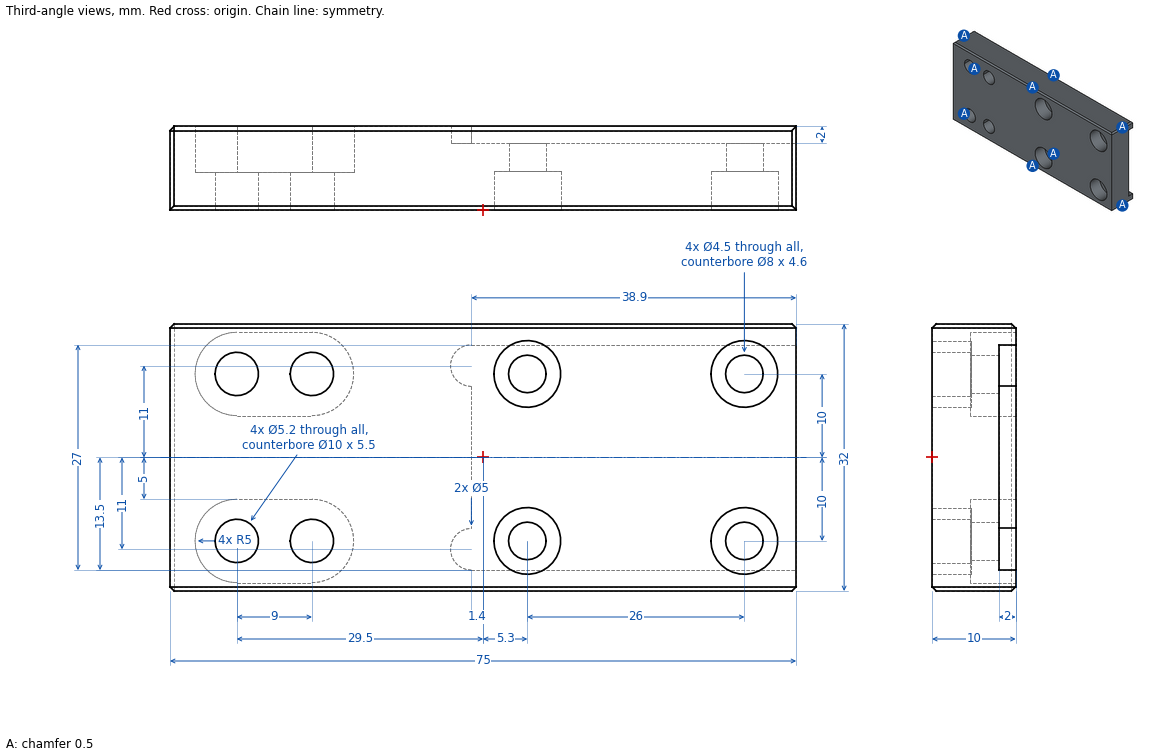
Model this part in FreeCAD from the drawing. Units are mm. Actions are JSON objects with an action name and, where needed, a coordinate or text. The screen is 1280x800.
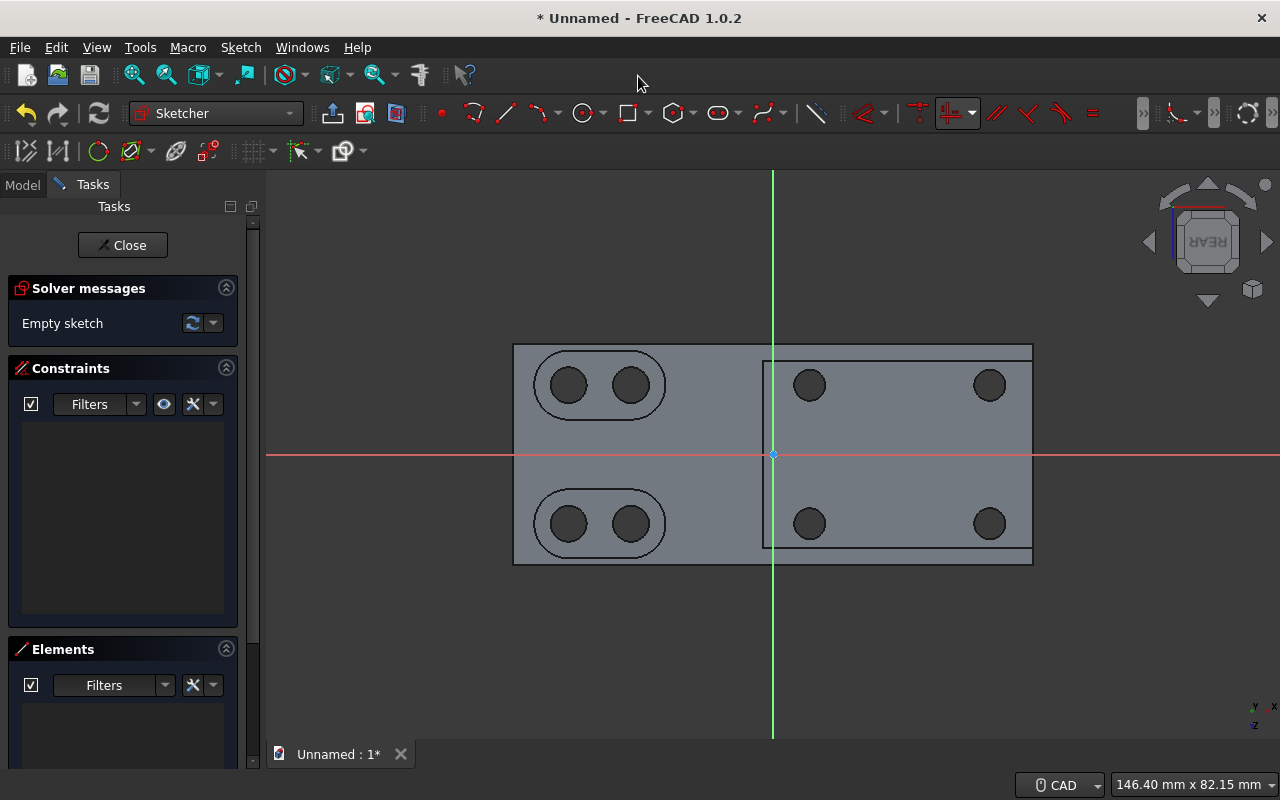
{"action": "scroll", "coordinate": [835, 454], "scroll_direction": "up", "scroll_amount": 3}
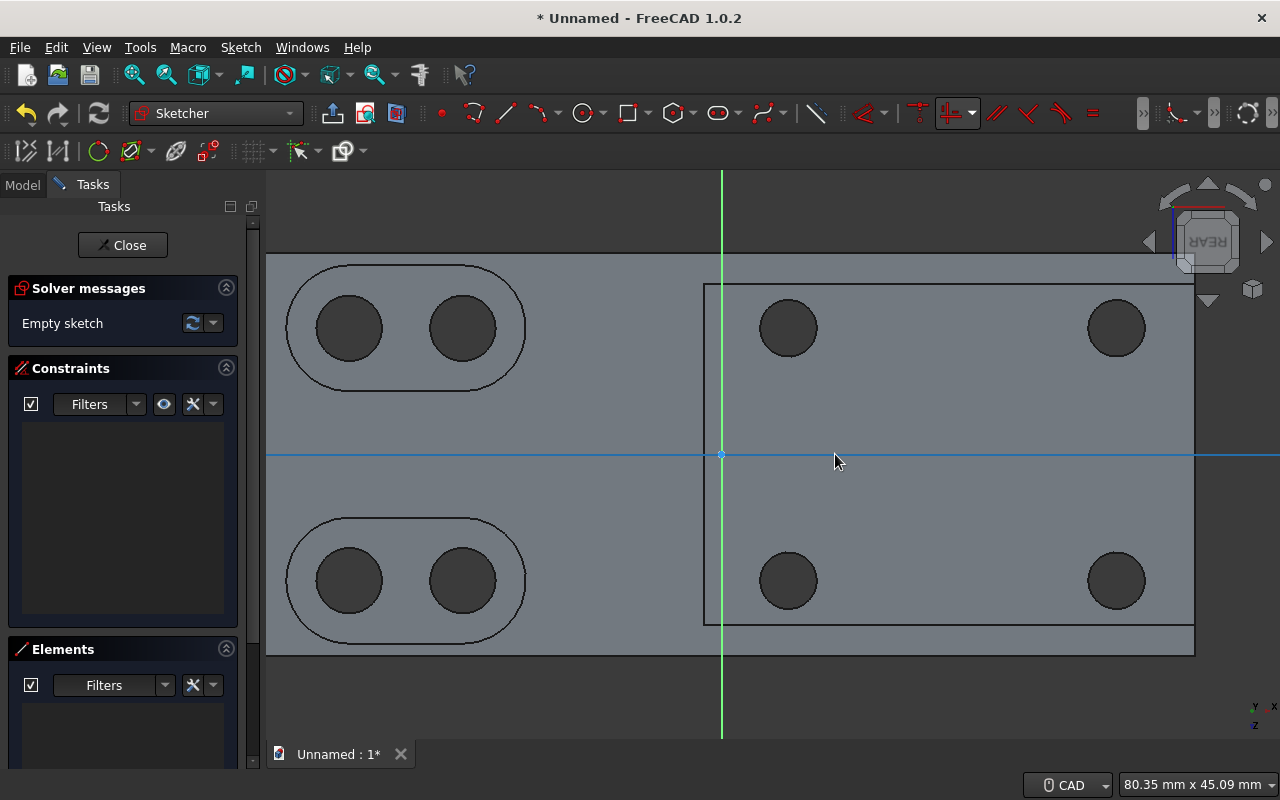
{"action": "left_click", "coordinate": [584, 114]}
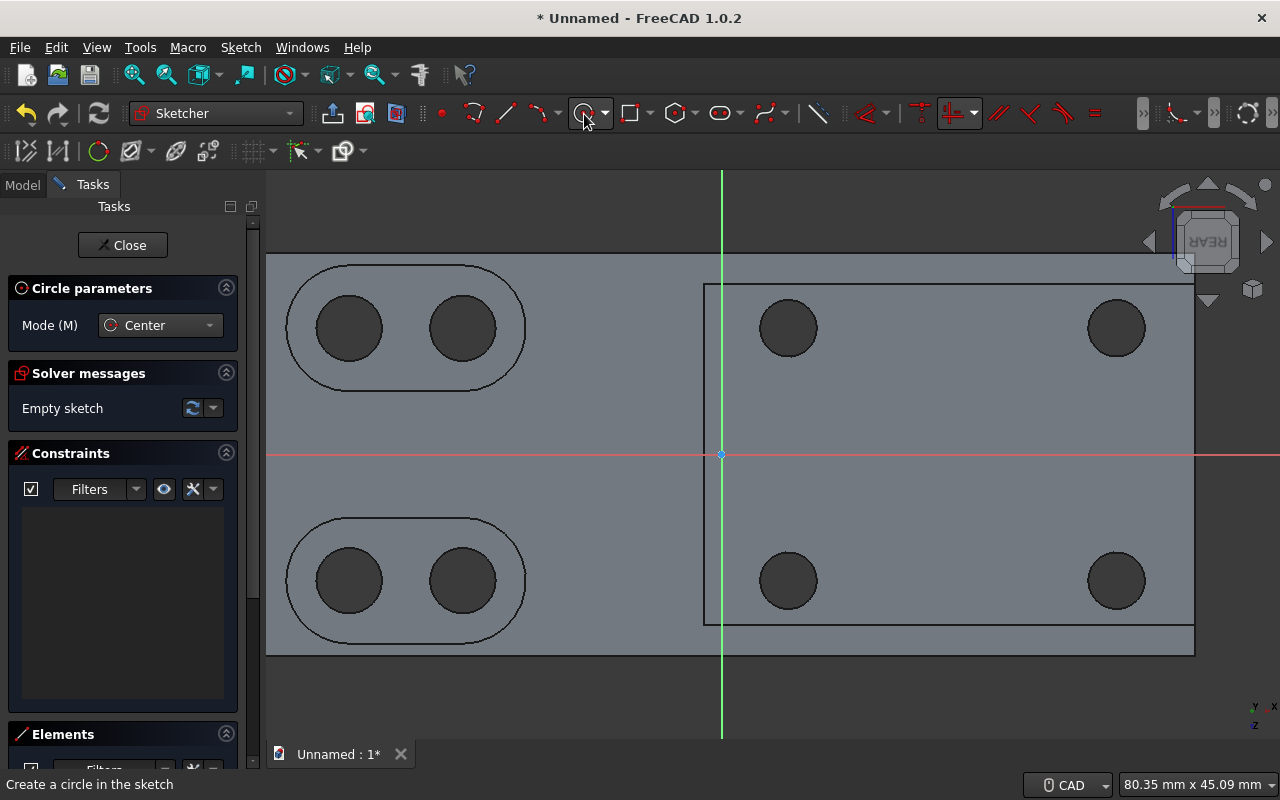
{"action": "left_click", "coordinate": [704, 316]}
{"action": "left_click", "coordinate": [682, 293]}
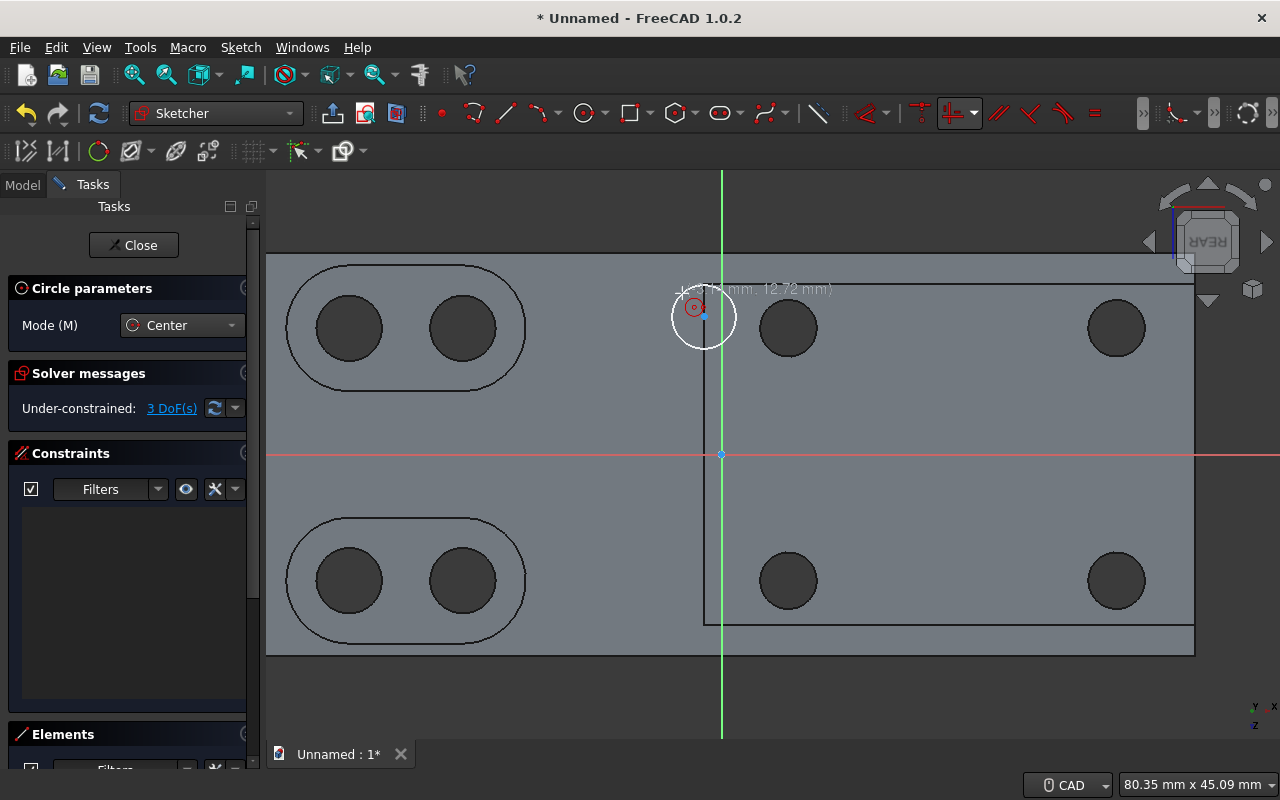
{"action": "left_click", "coordinate": [704, 593]}
{"action": "left_click", "coordinate": [682, 571]}
{"action": "key", "text": "Escape"}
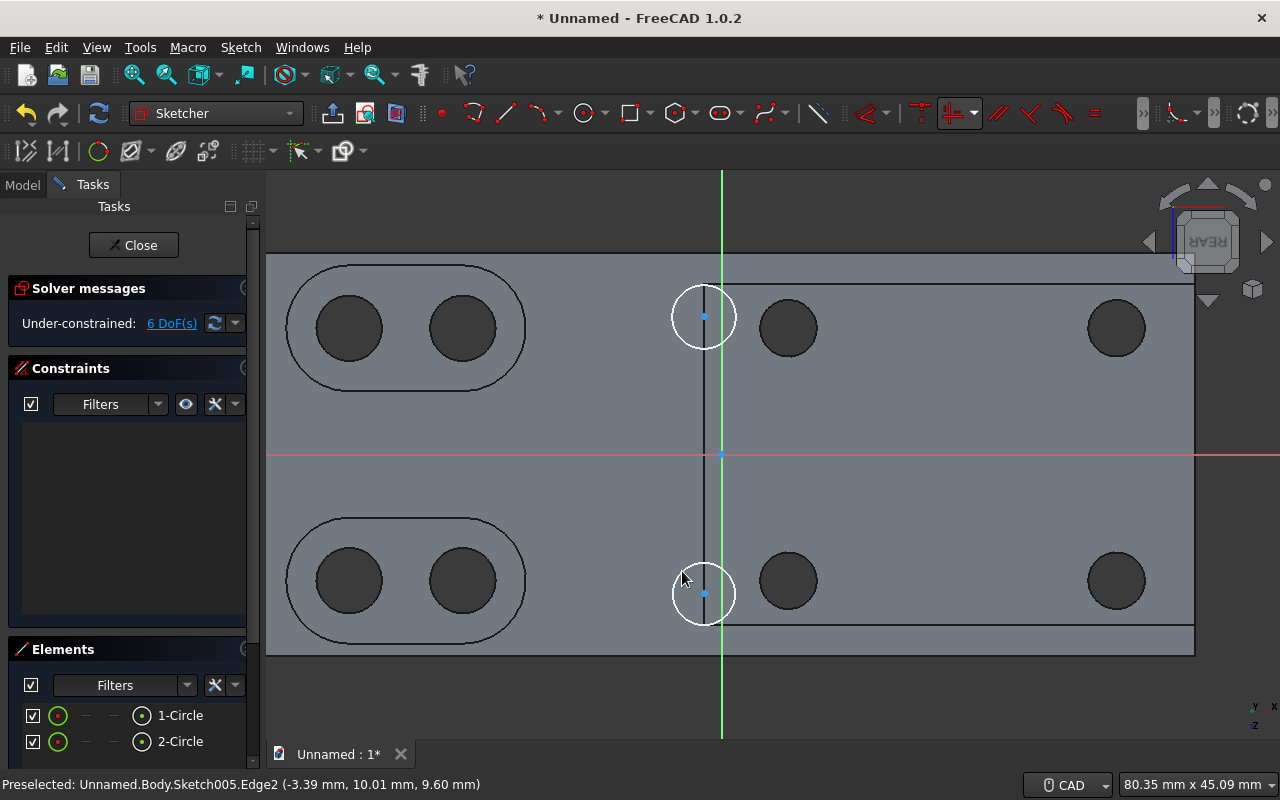
{"action": "left_click", "coordinate": [681, 295]}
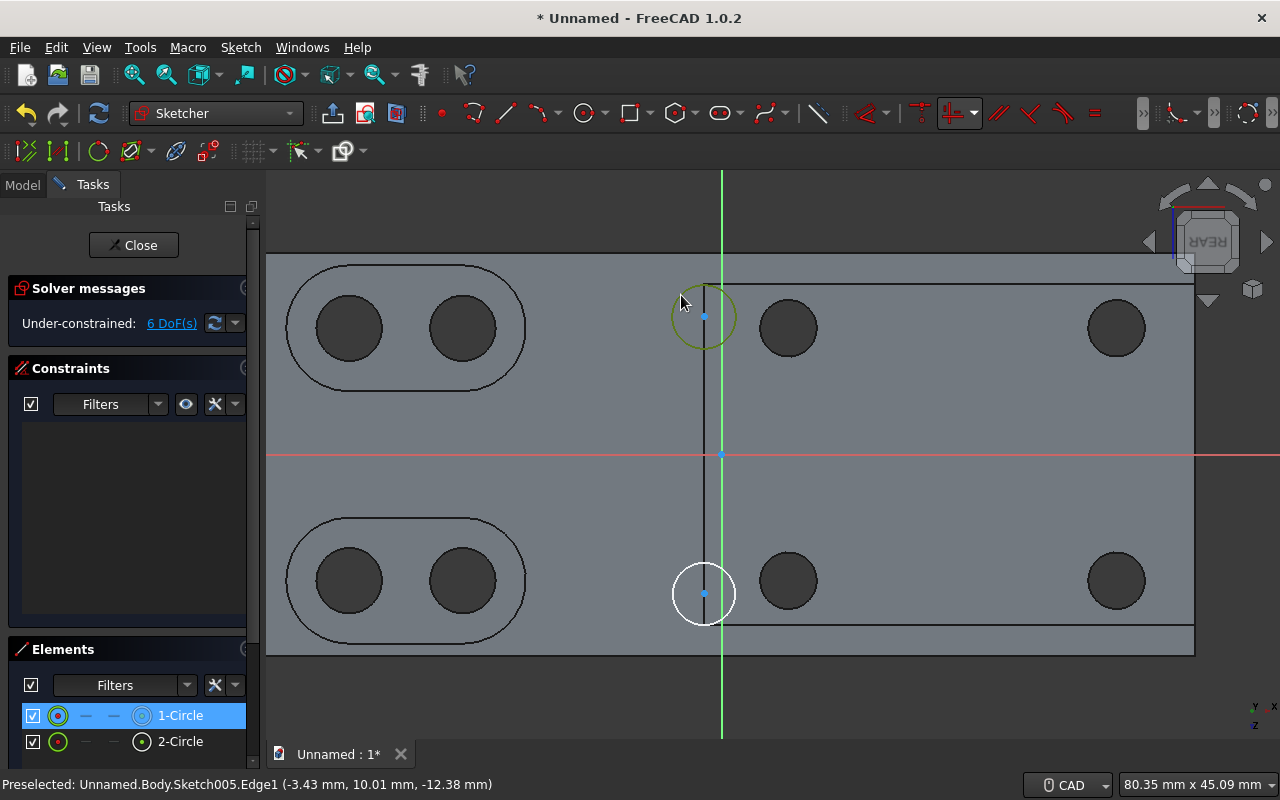
{"action": "left_click", "coordinate": [682, 572]}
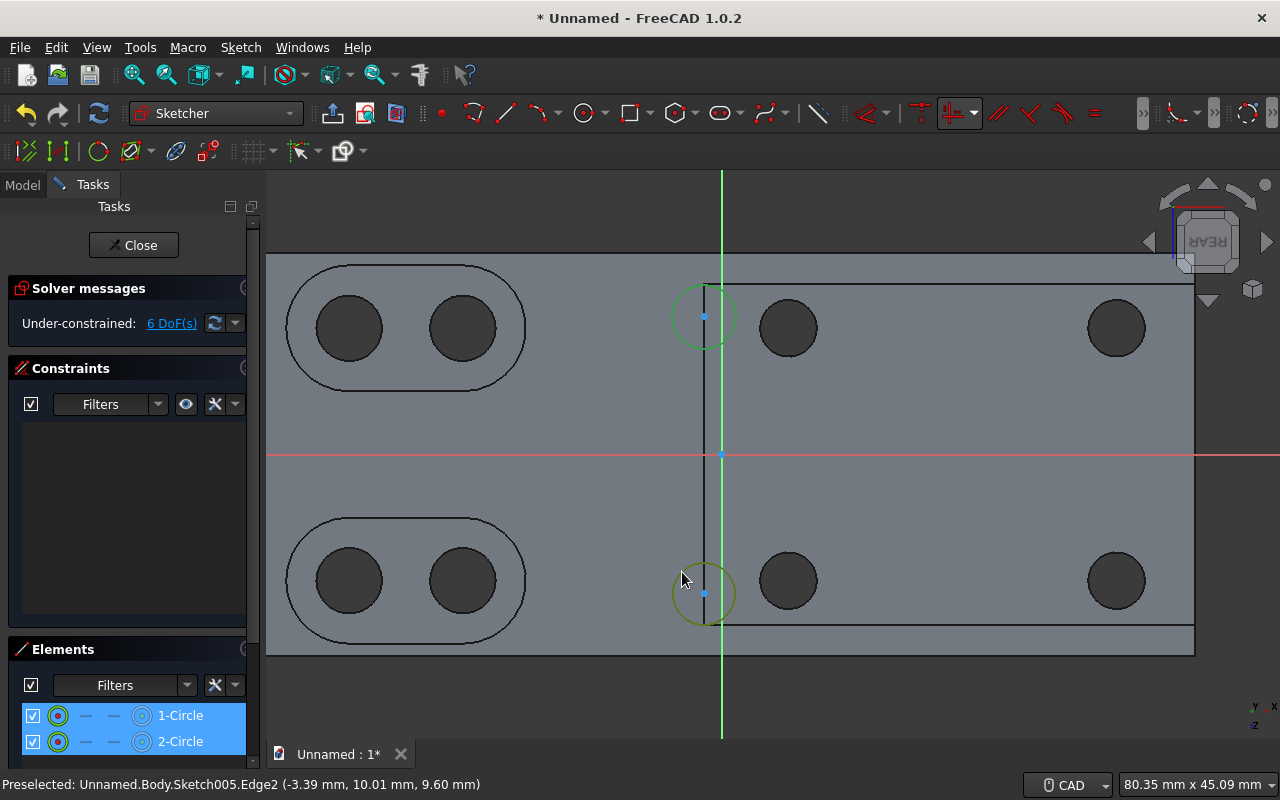
{"action": "left_click", "coordinate": [1096, 114]}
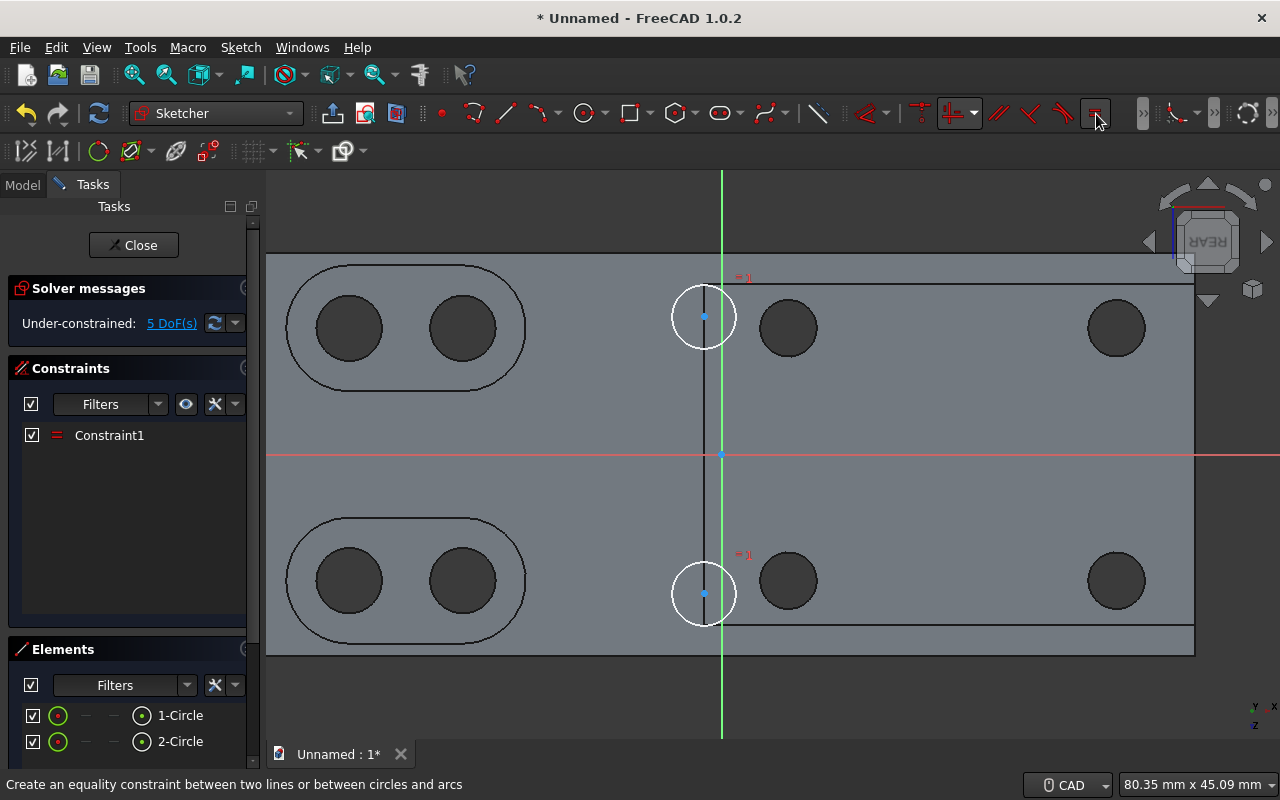
{"action": "left_click", "coordinate": [704, 317]}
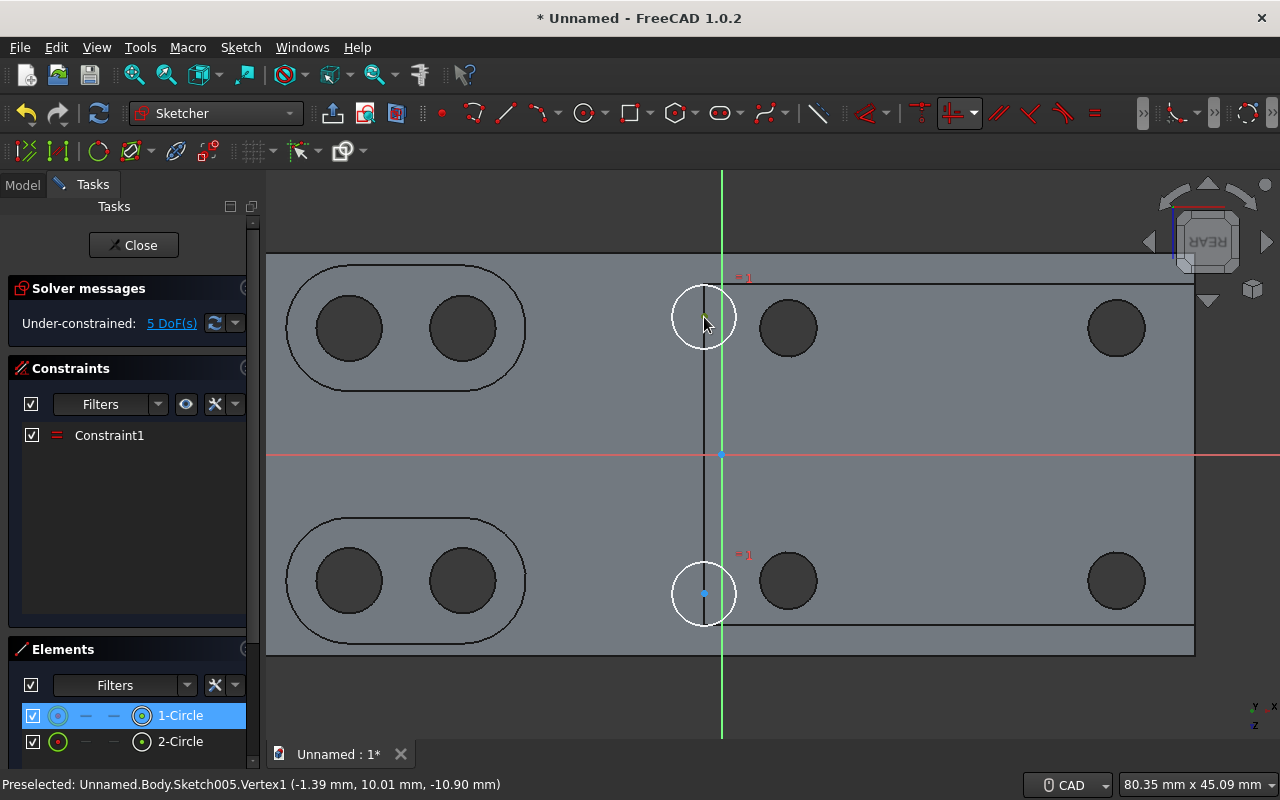
{"action": "left_click", "coordinate": [704, 594]}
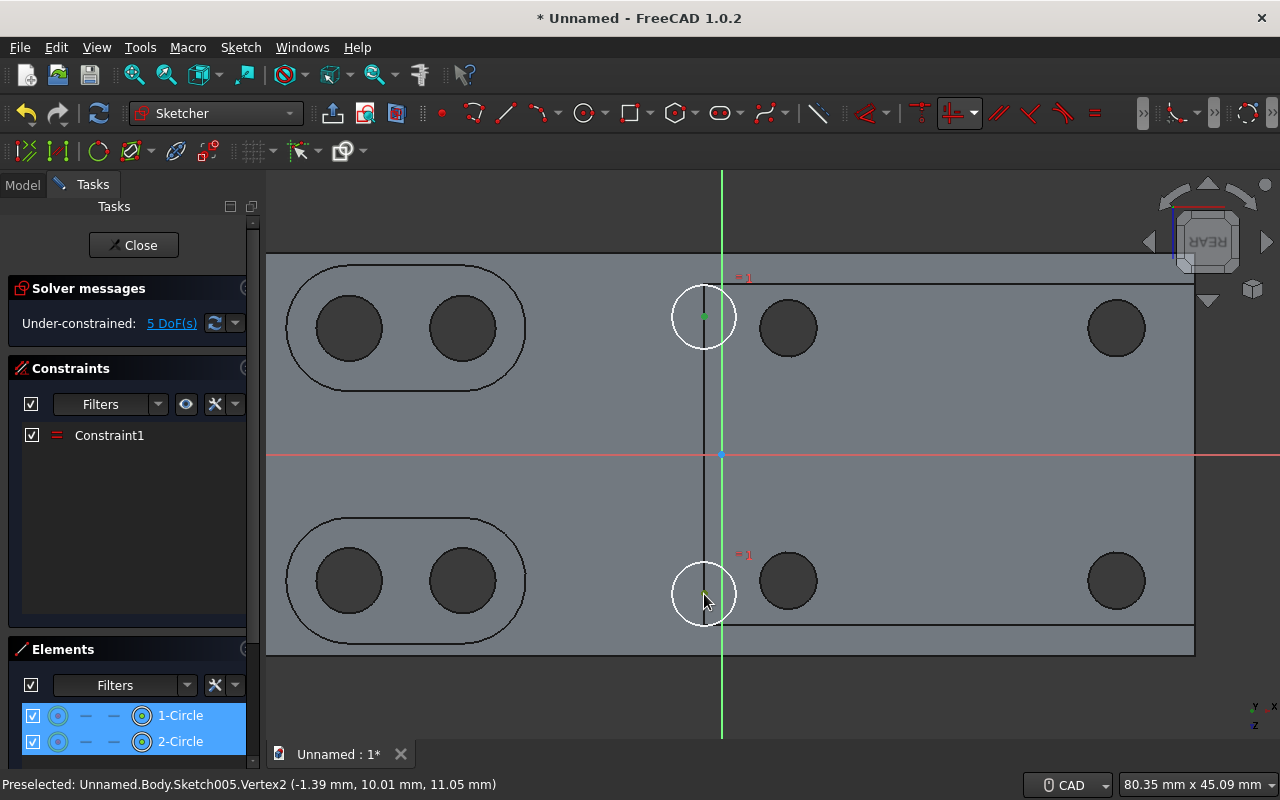
{"action": "left_click", "coordinate": [976, 114]}